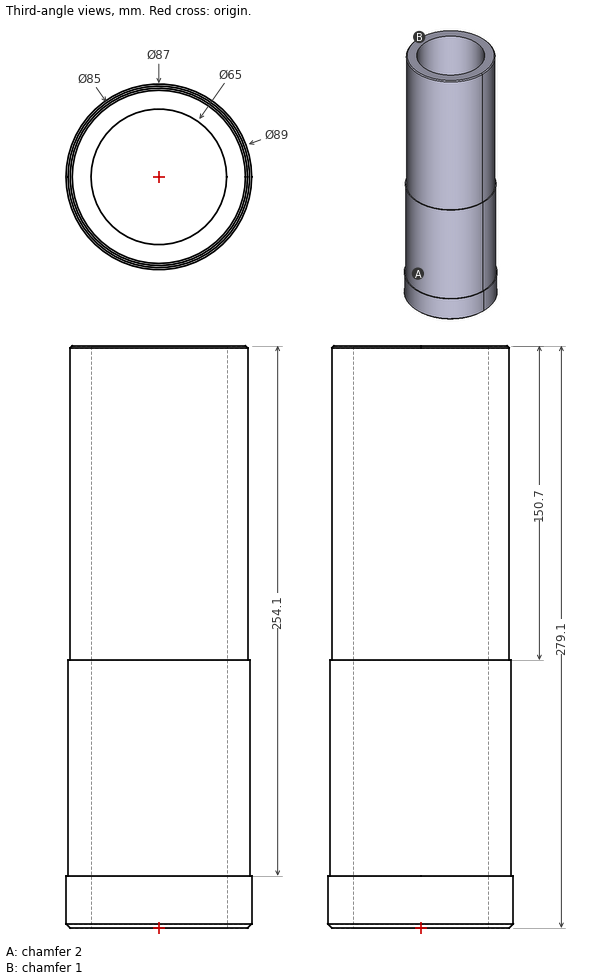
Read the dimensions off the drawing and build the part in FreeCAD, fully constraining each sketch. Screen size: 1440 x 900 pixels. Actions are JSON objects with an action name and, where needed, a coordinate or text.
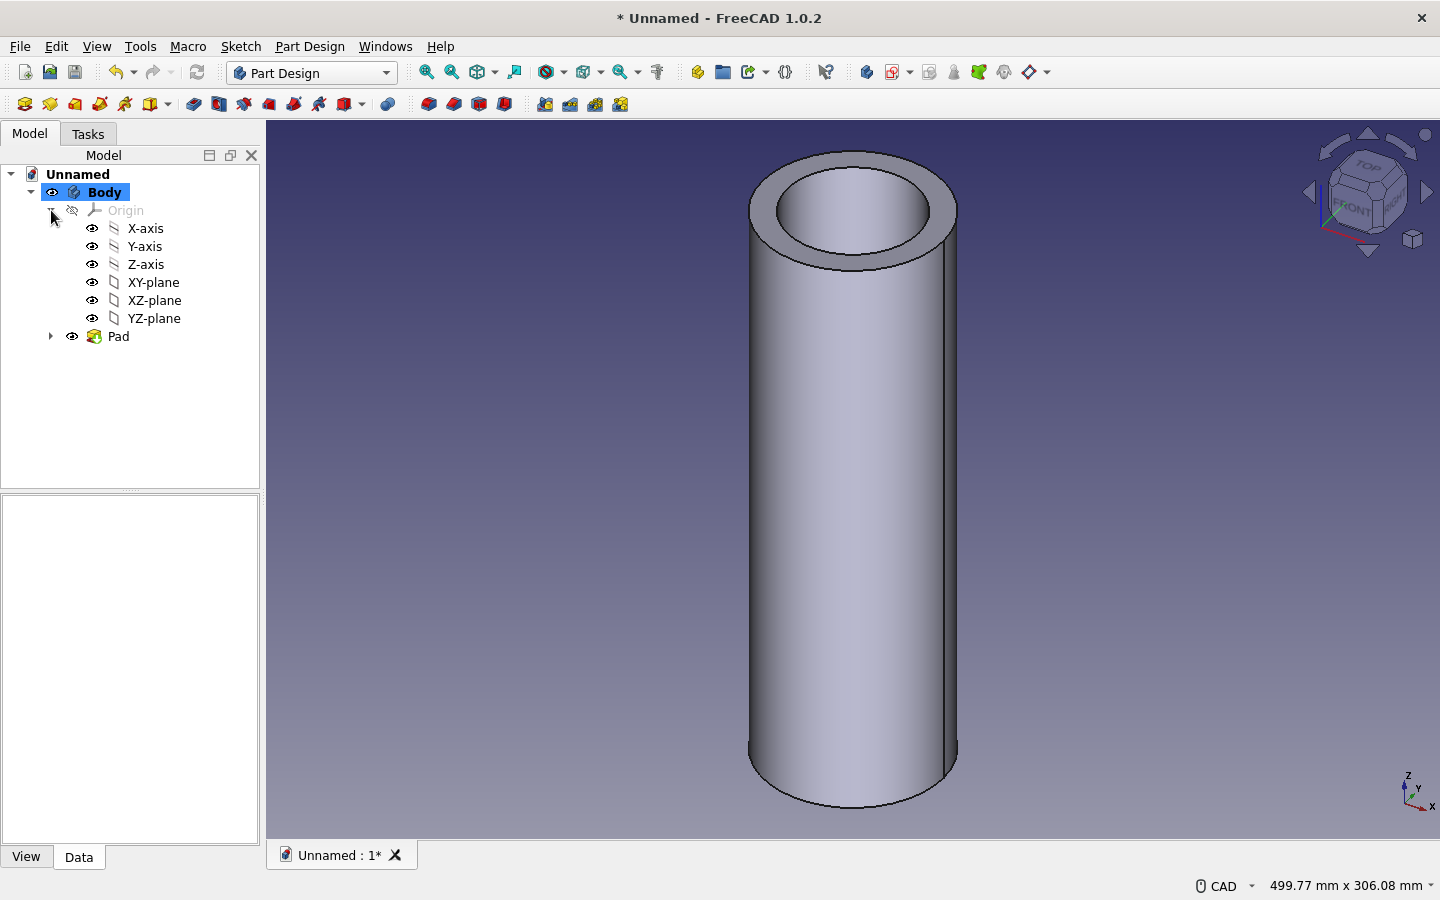
{"action": "left_click", "coordinate": [137, 282]}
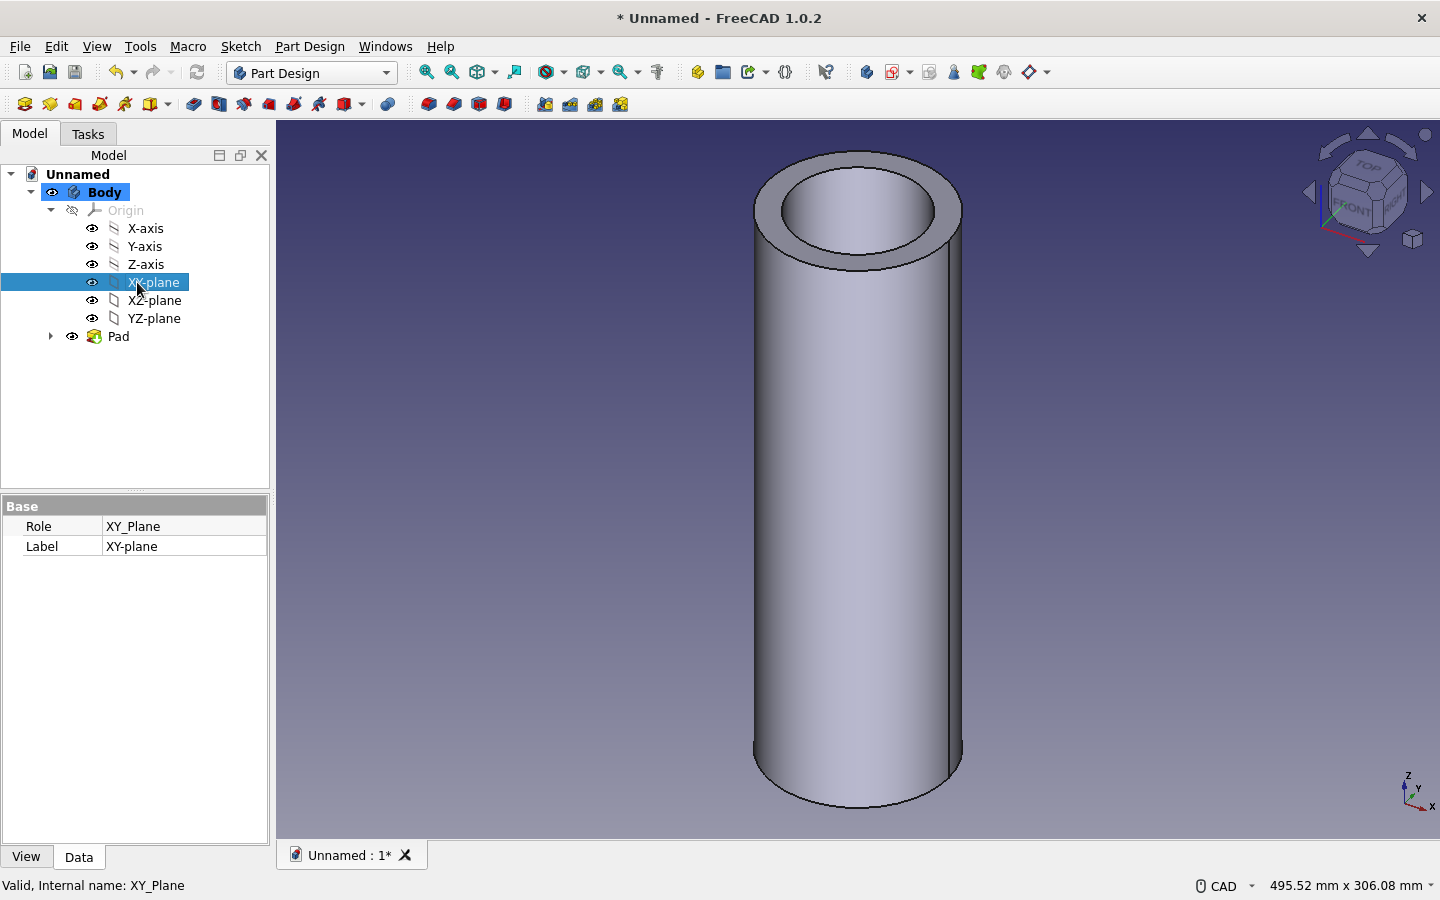
{"action": "left_click", "coordinate": [1028, 72]}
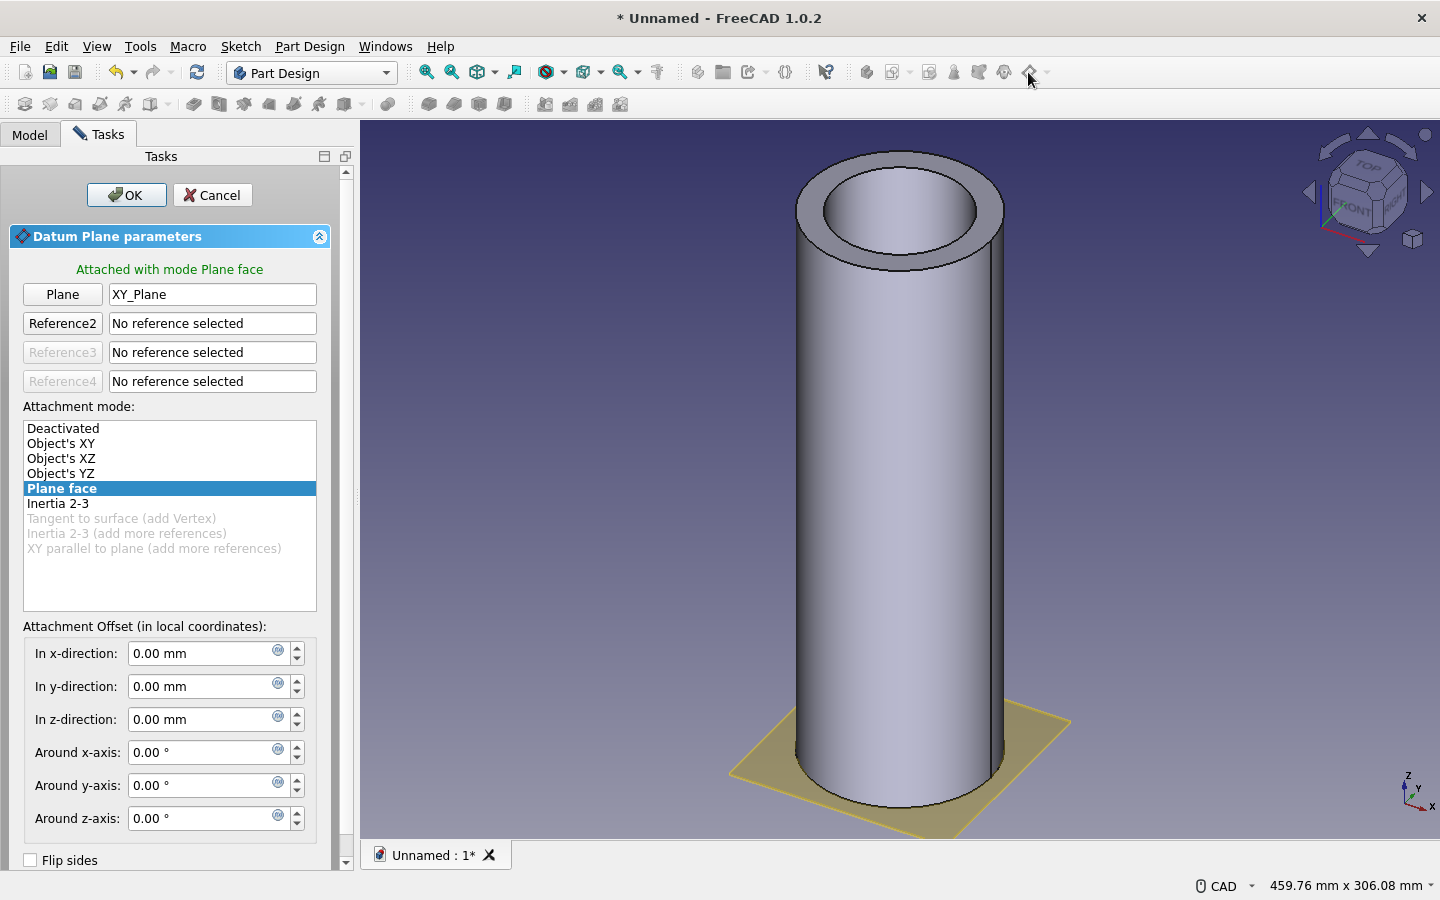
{"action": "triple_click", "coordinate": [210, 720]}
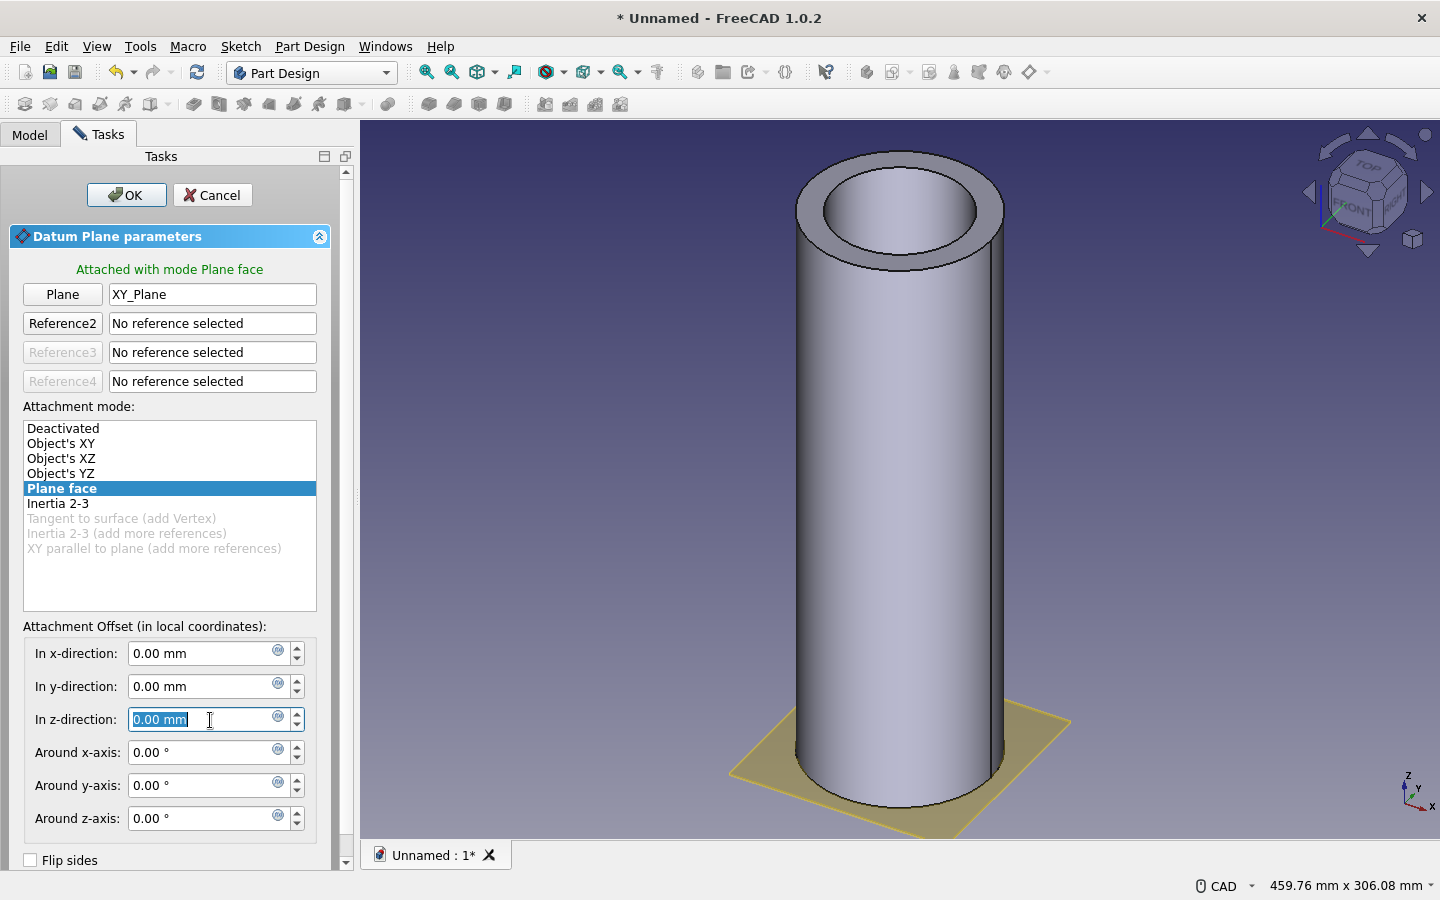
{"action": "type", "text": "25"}
{"action": "key", "text": "Tab"}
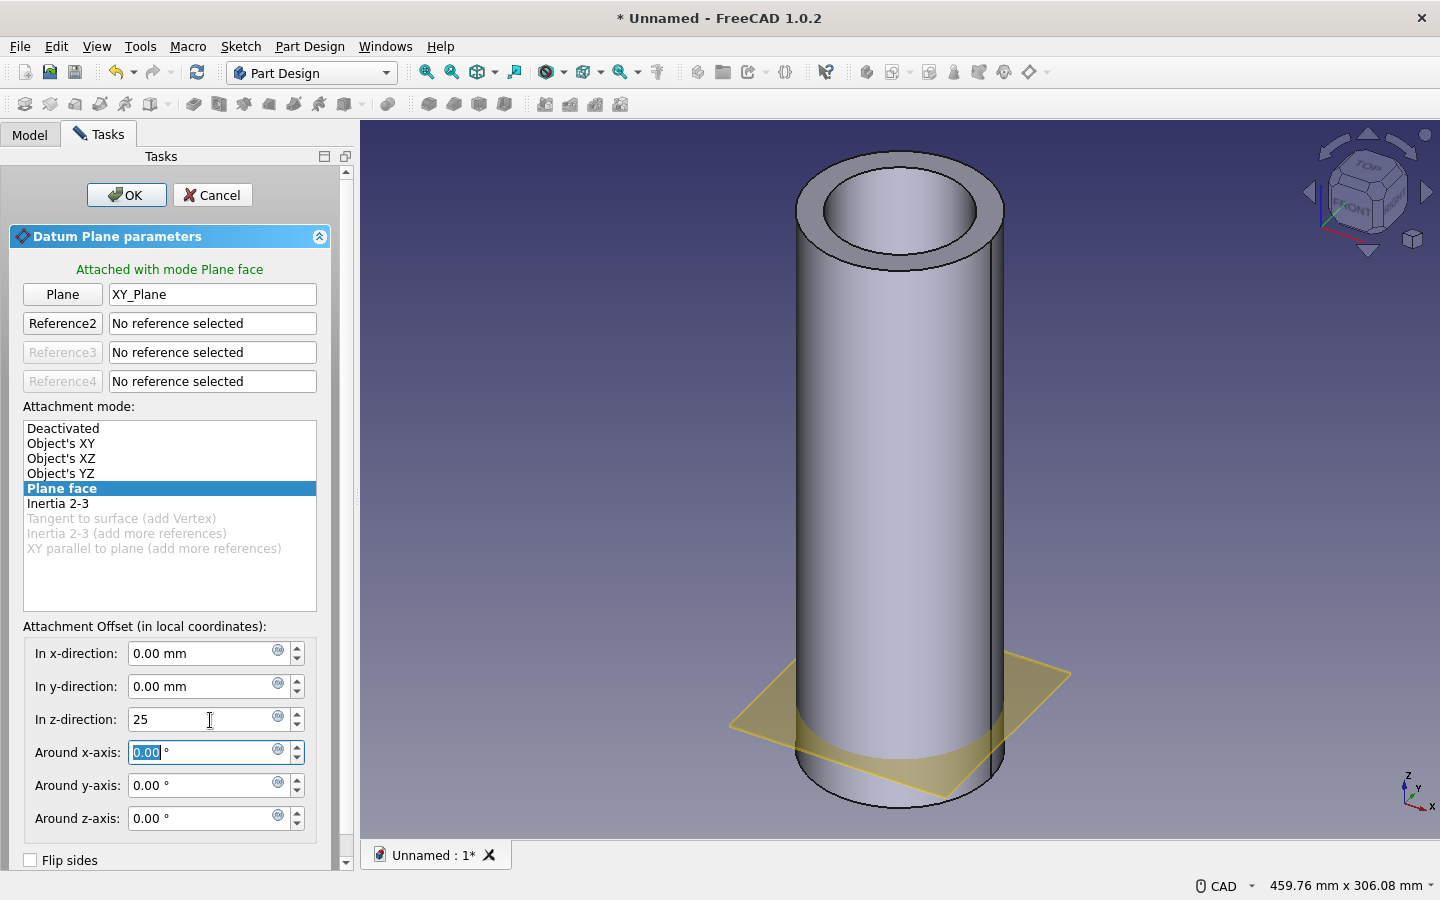
{"action": "left_click", "coordinate": [127, 195]}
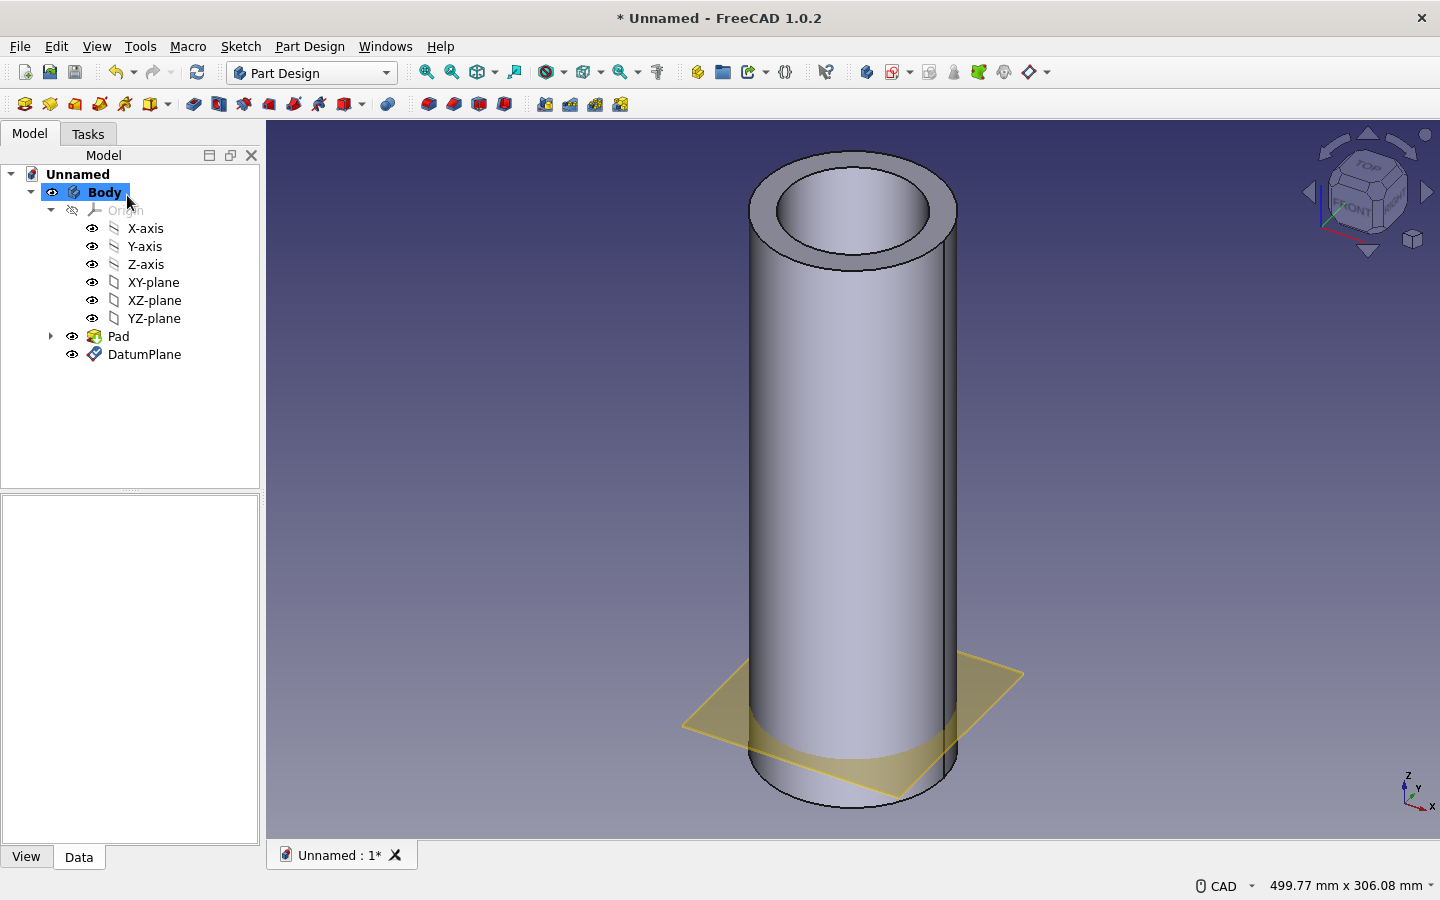
{"action": "left_click", "coordinate": [117, 354]}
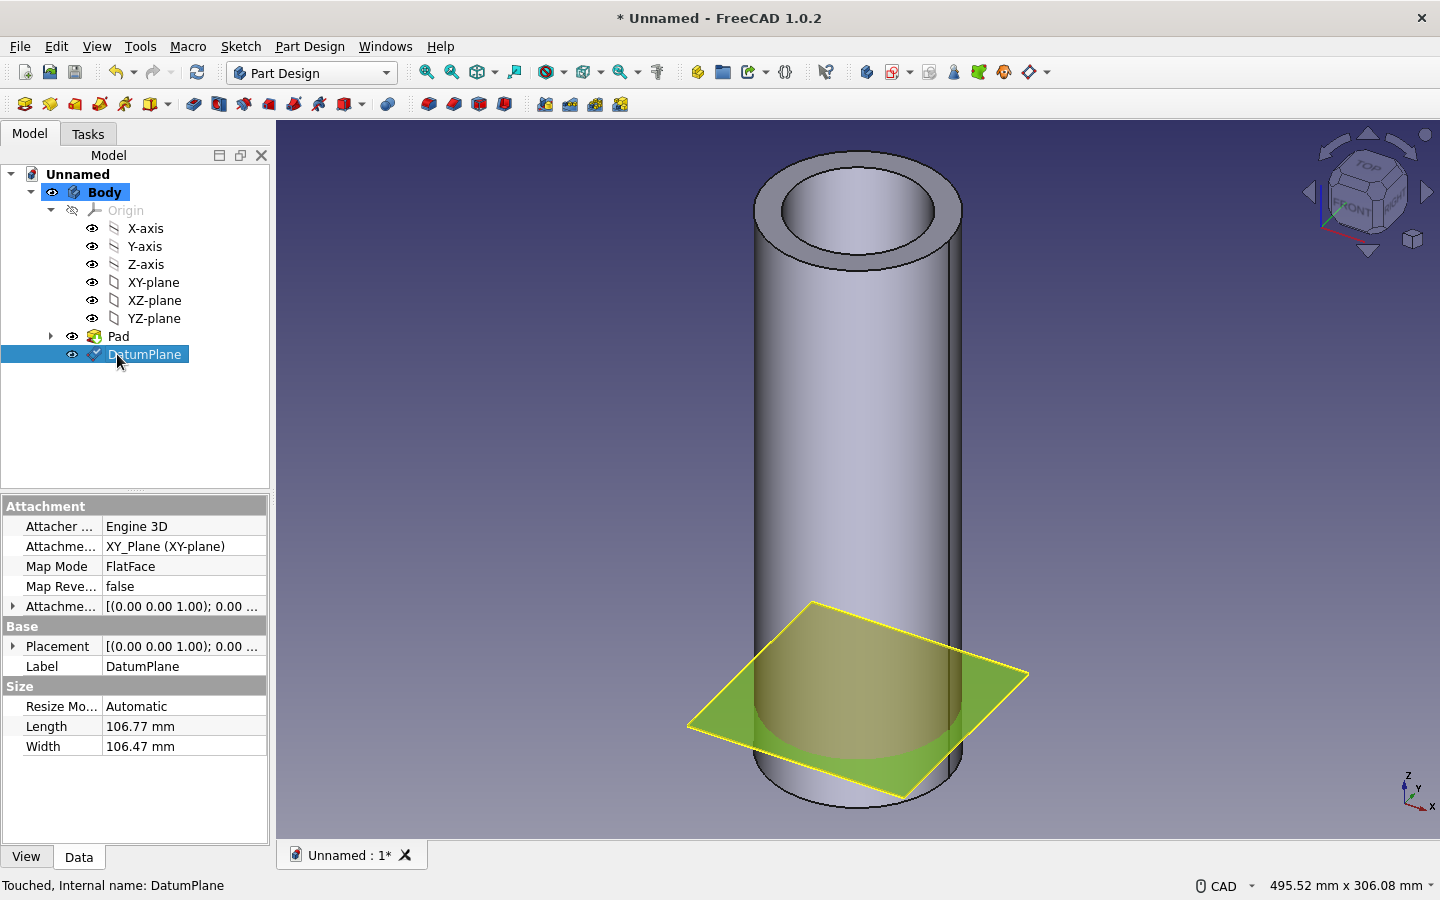
{"action": "left_click", "coordinate": [892, 72]}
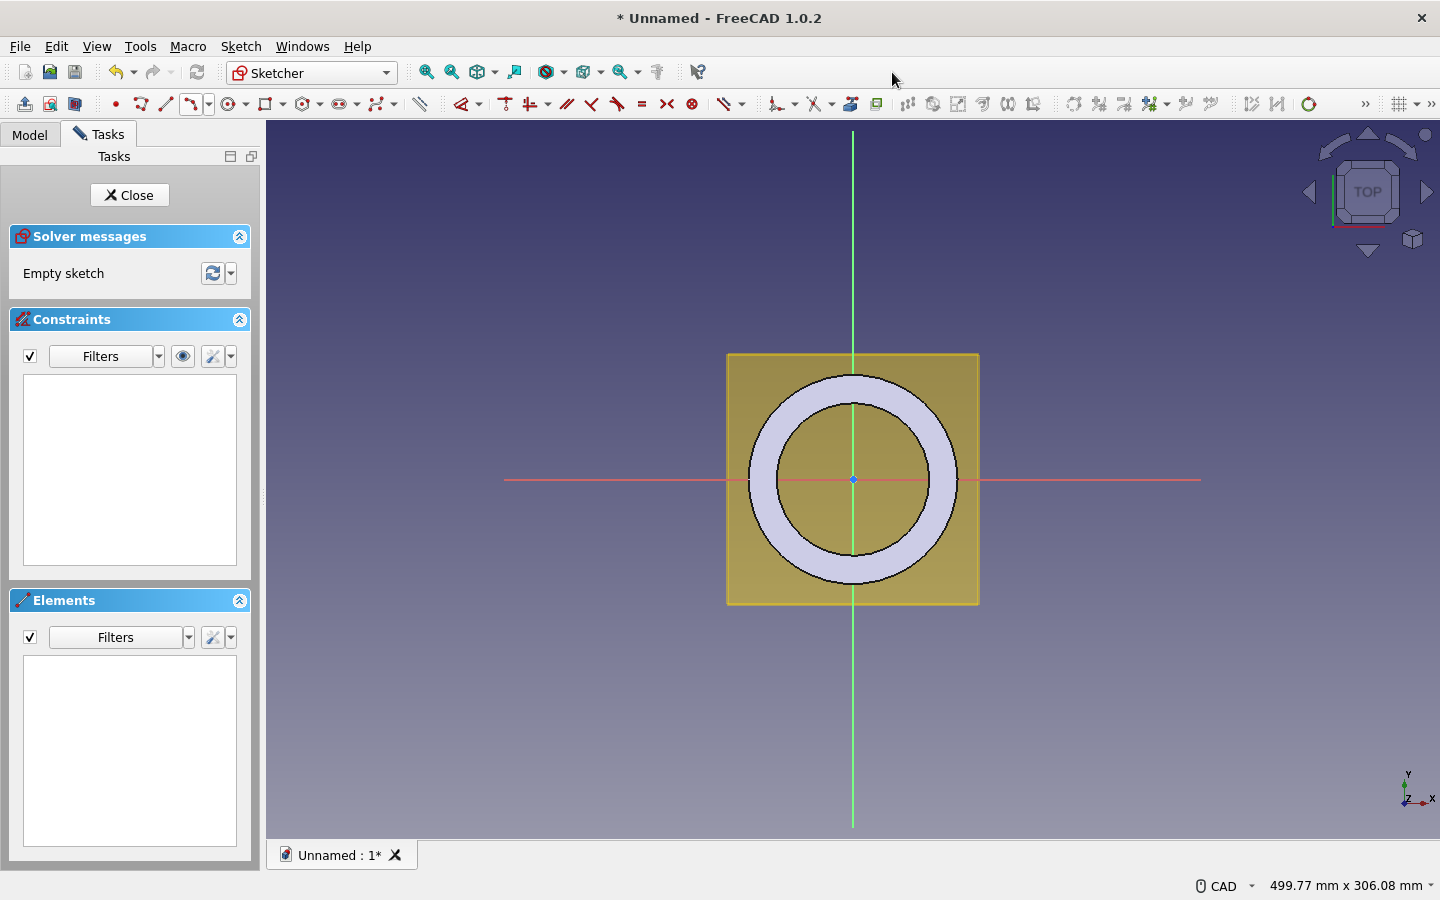
{"action": "key", "text": "q s"}